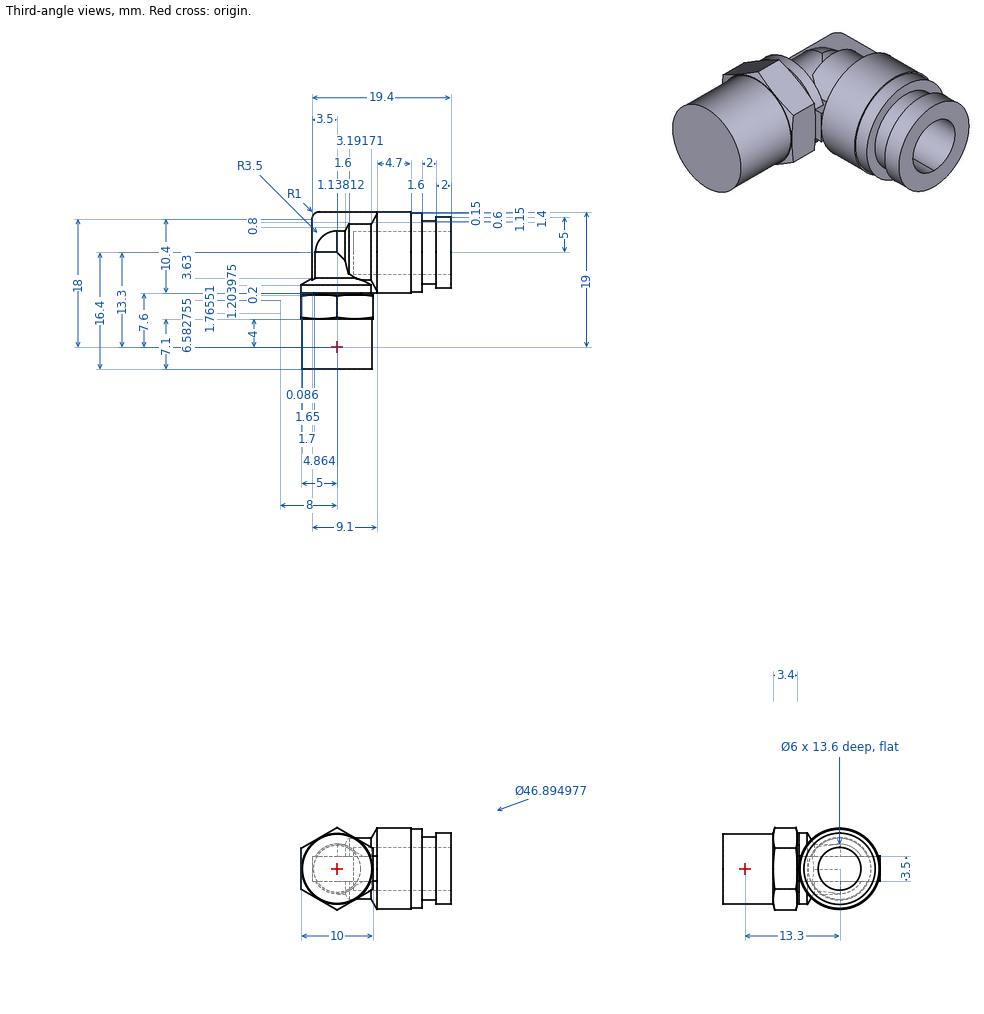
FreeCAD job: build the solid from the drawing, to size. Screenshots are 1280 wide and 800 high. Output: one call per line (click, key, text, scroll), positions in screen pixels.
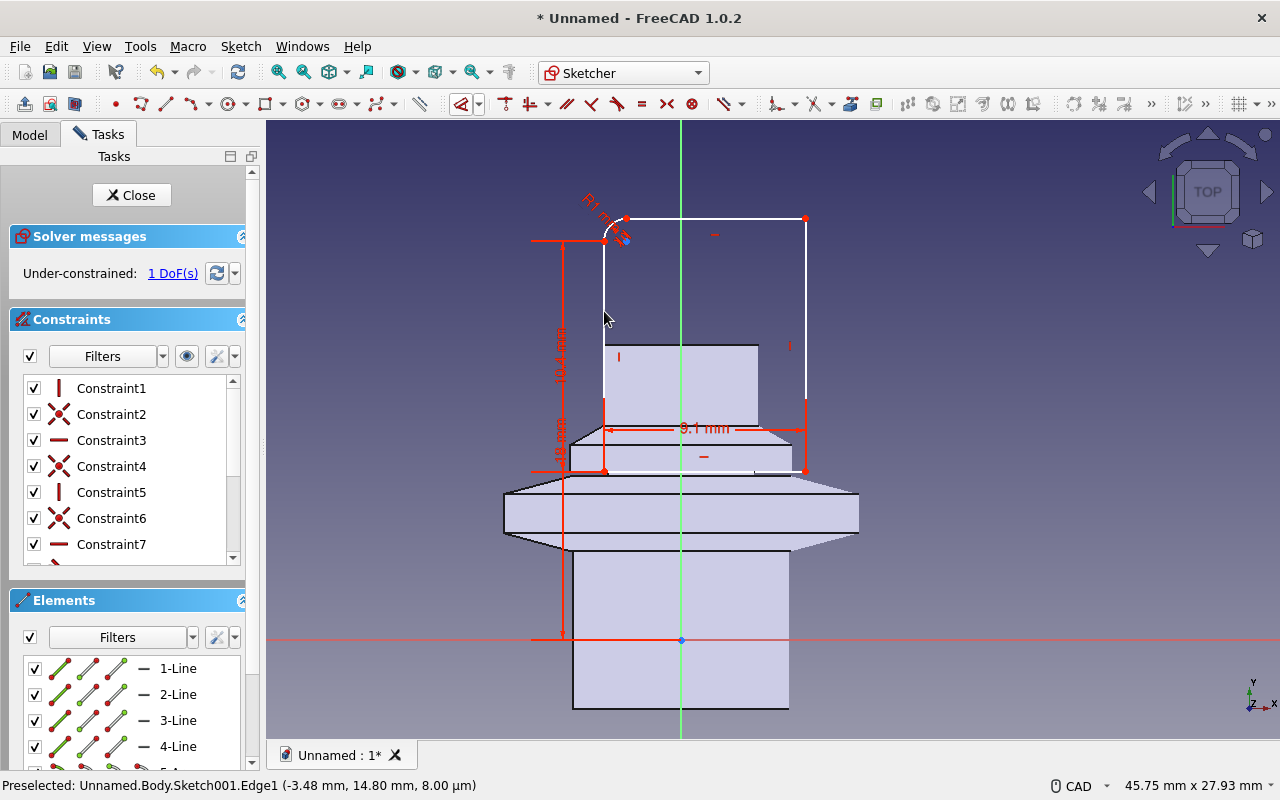
click(604, 241)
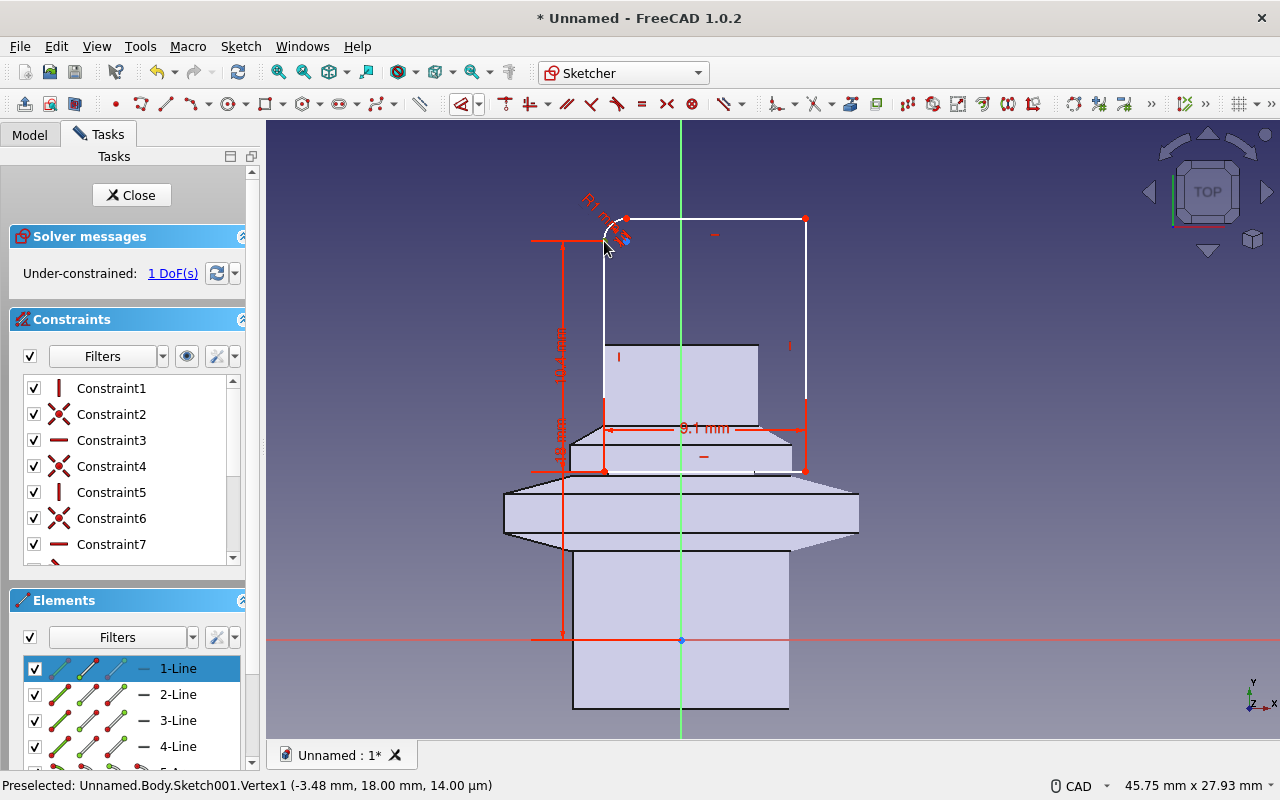
key(l)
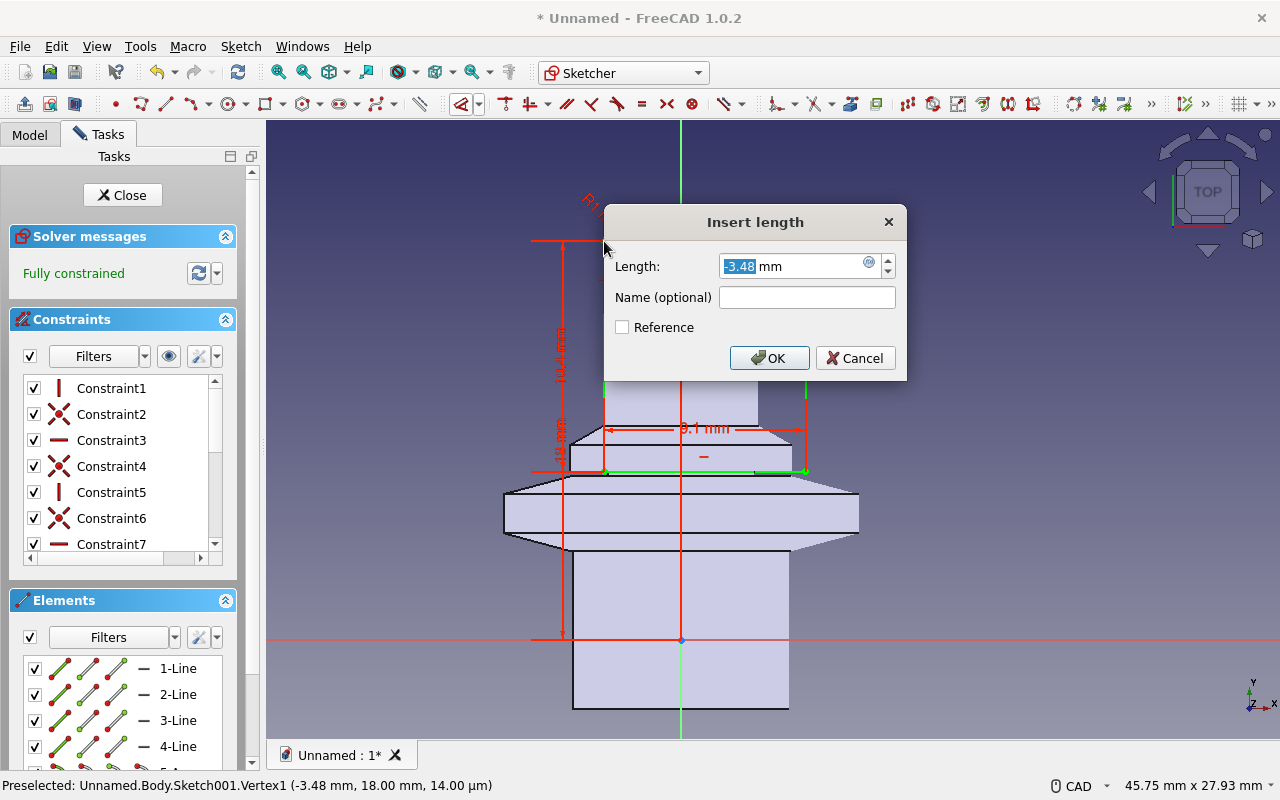
text(-3.5)
key(Return)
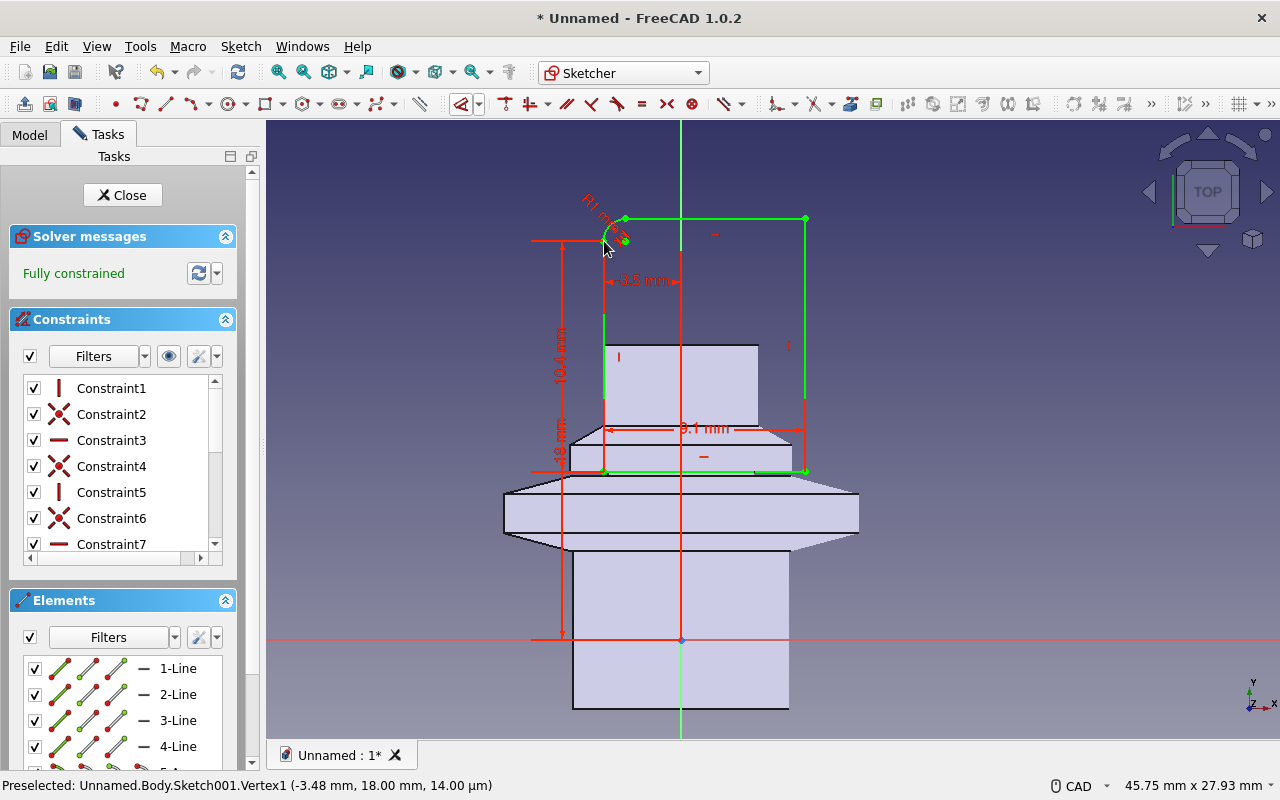
click(123, 195)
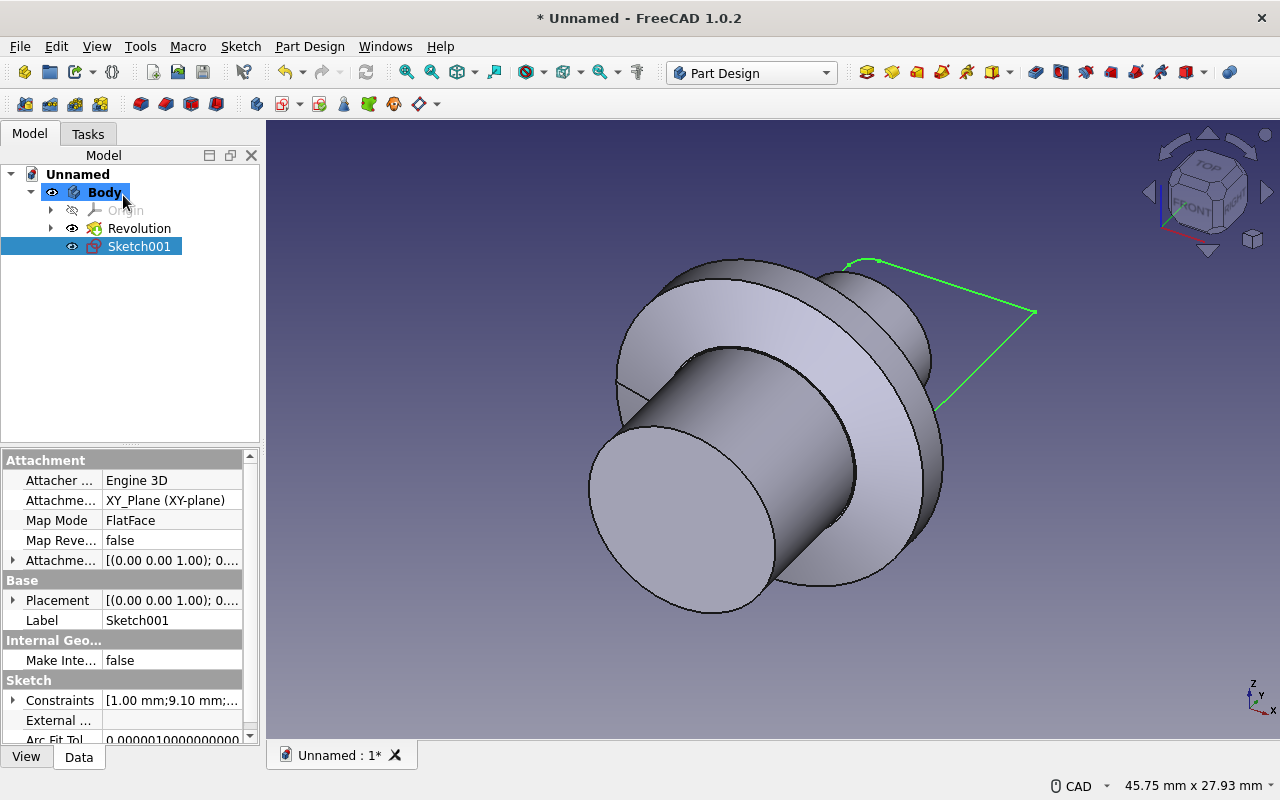
click(867, 72)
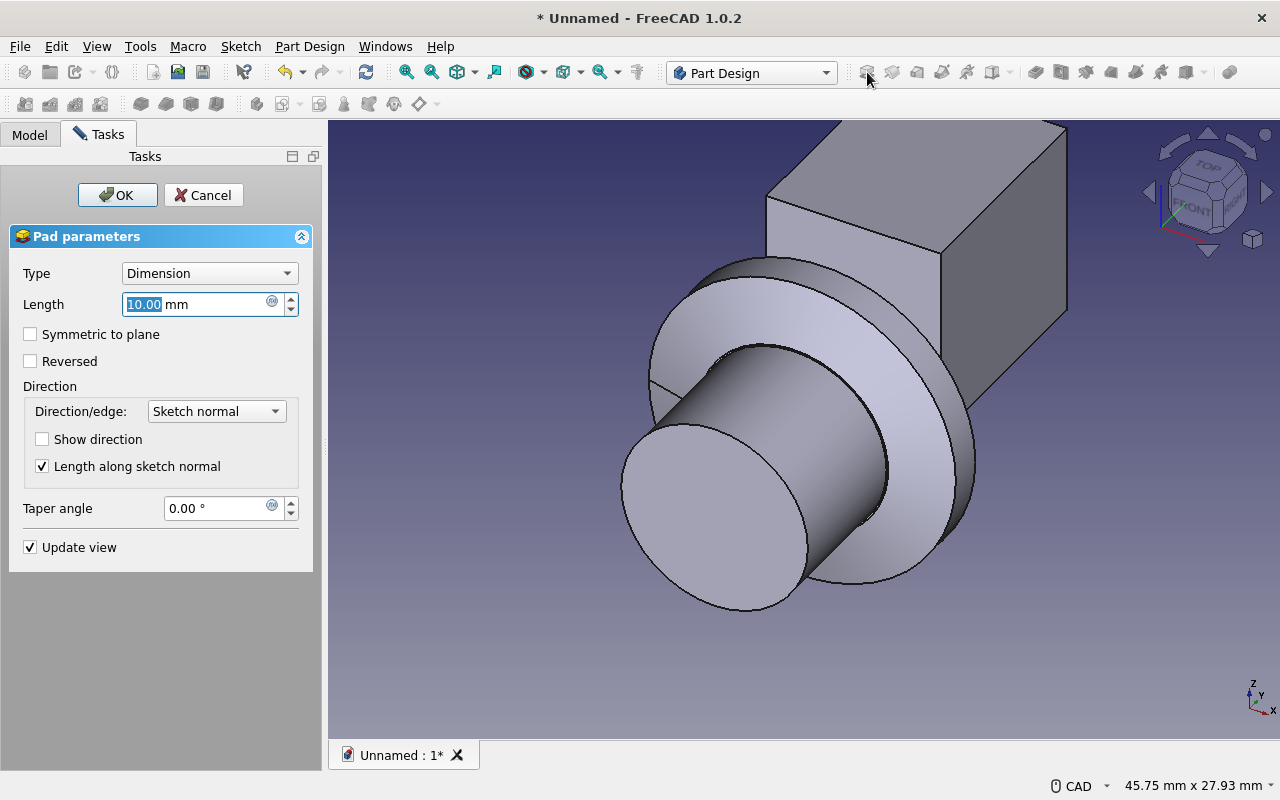
text(3.5)
key(Tab)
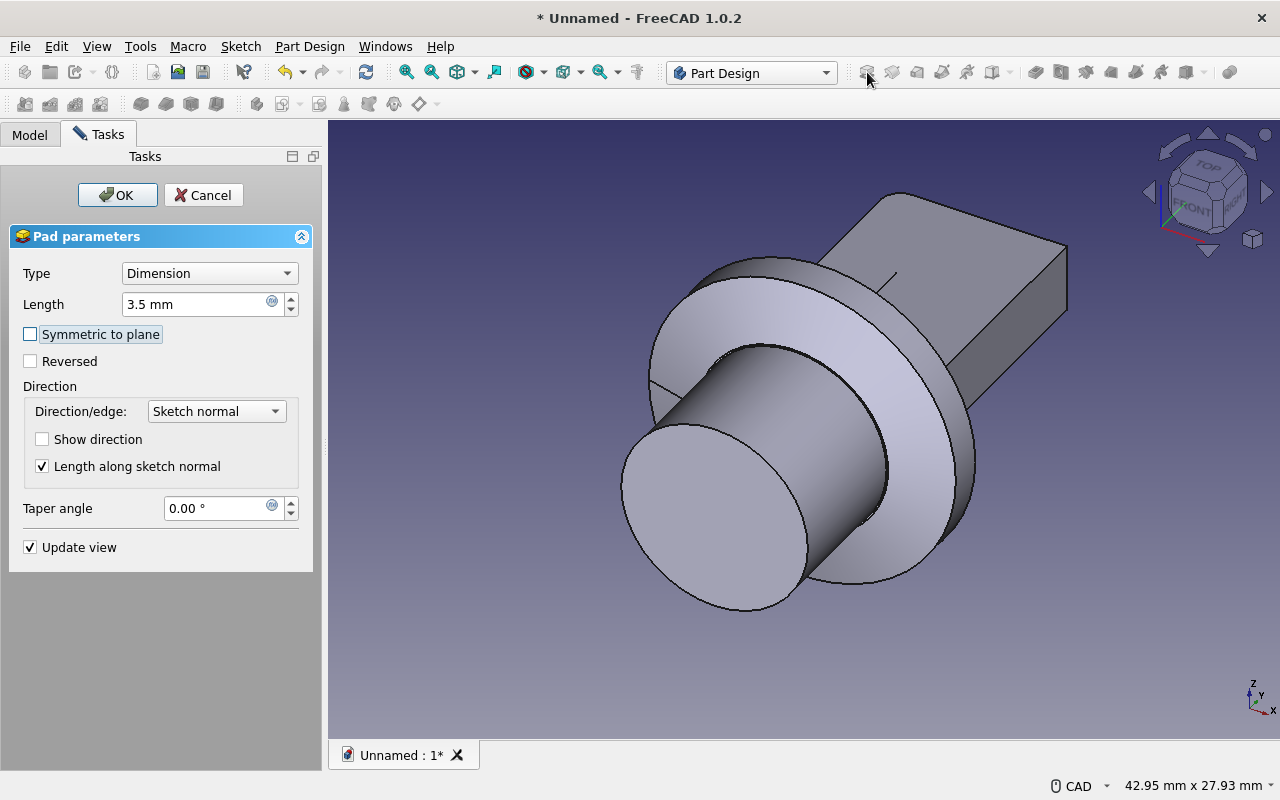
click(31, 334)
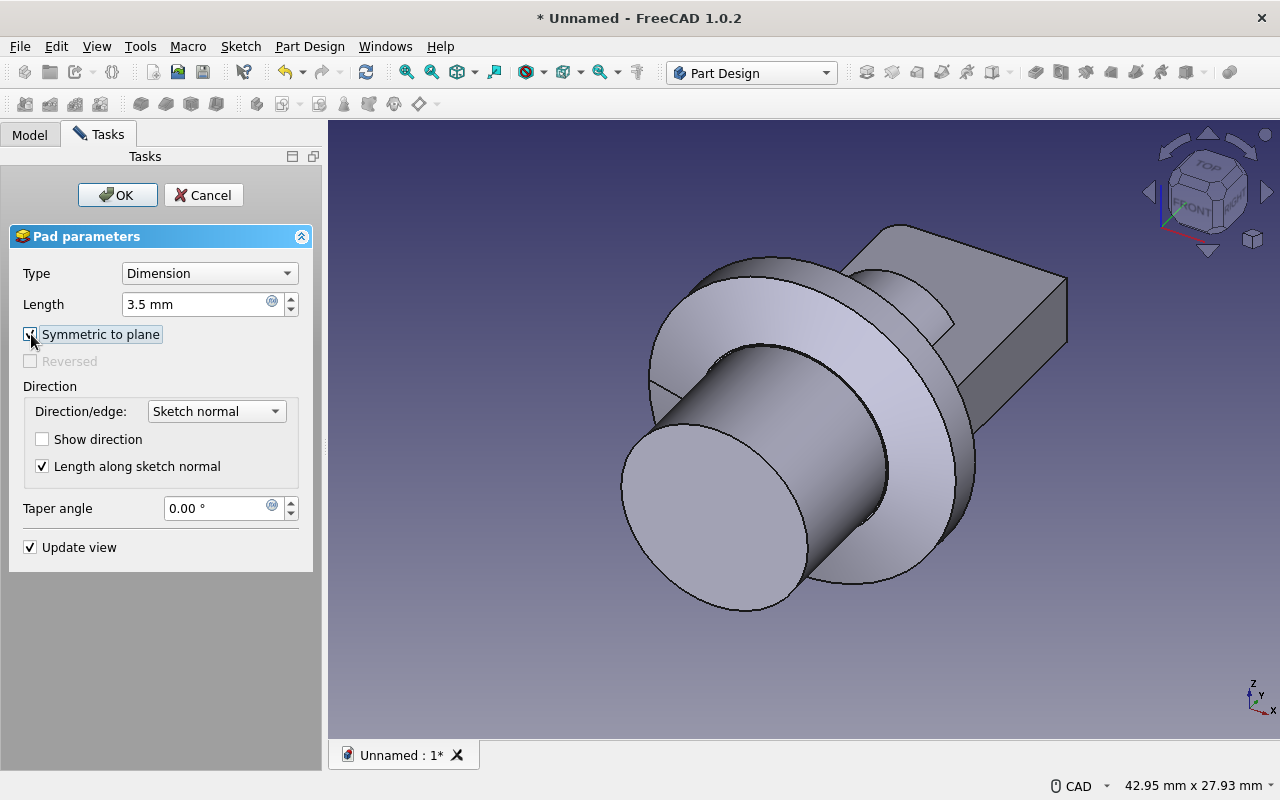
click(118, 195)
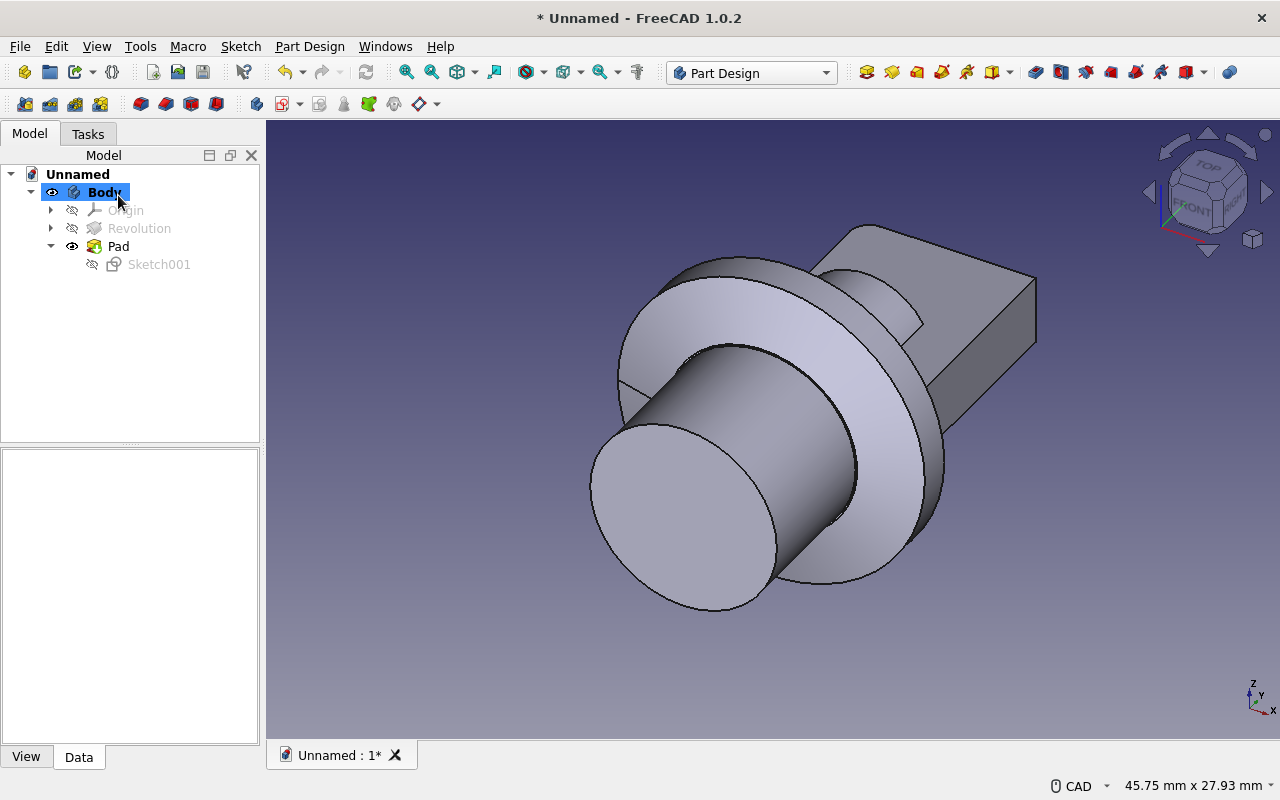
key(v)
key(f)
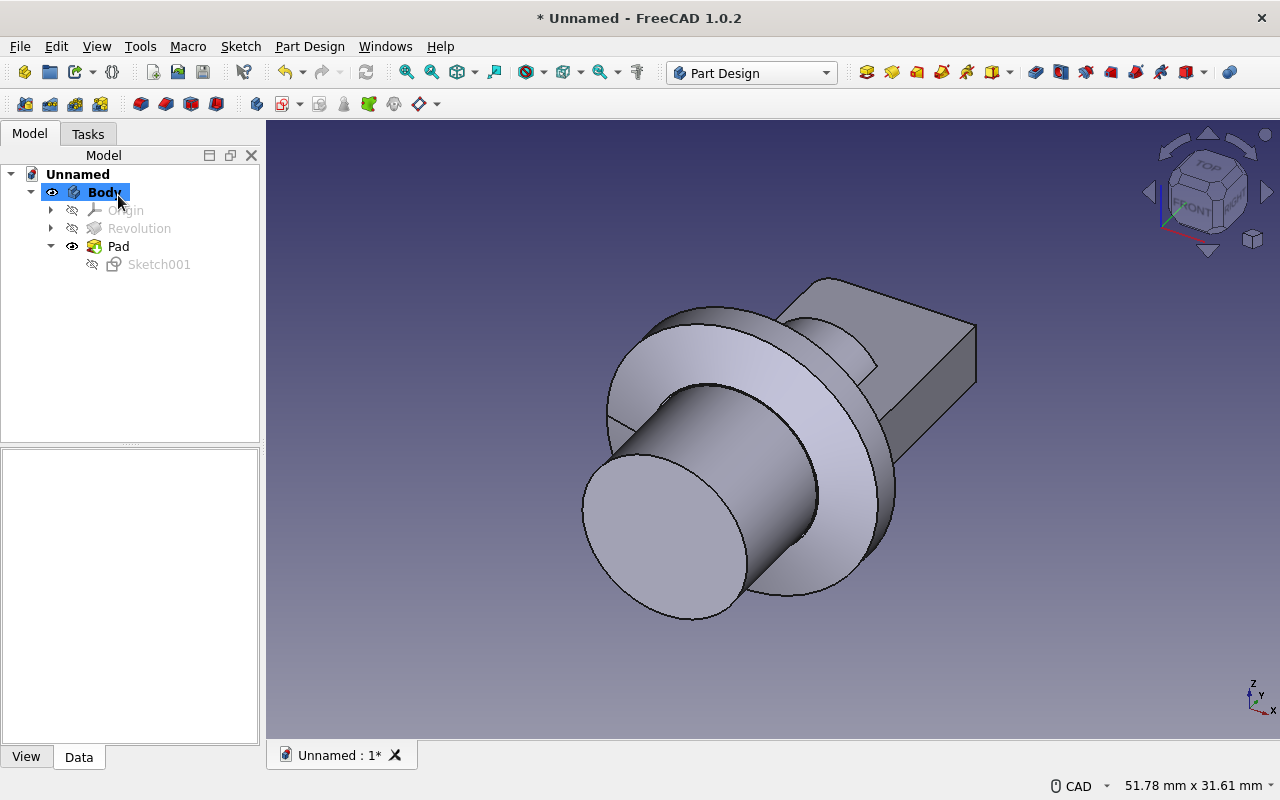
click(51, 210)